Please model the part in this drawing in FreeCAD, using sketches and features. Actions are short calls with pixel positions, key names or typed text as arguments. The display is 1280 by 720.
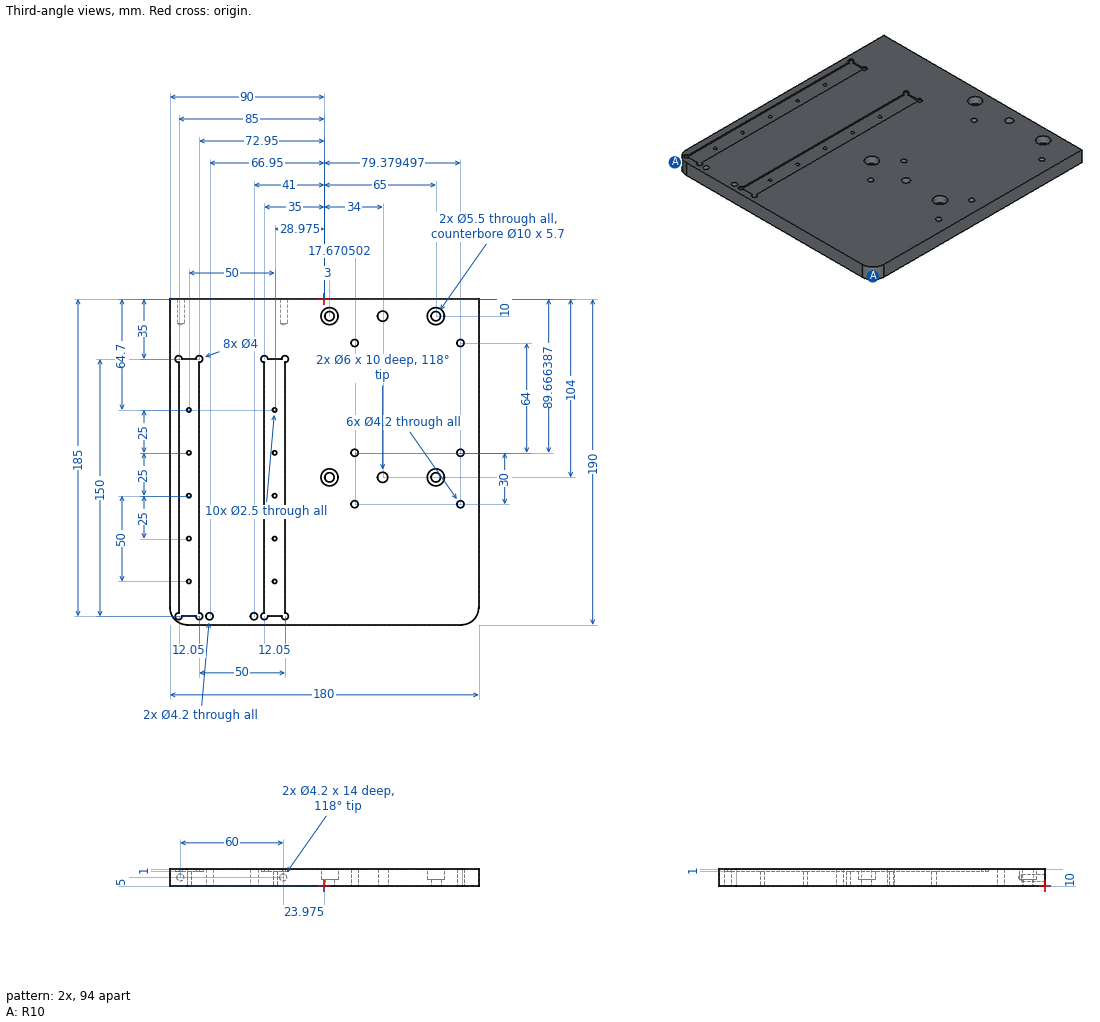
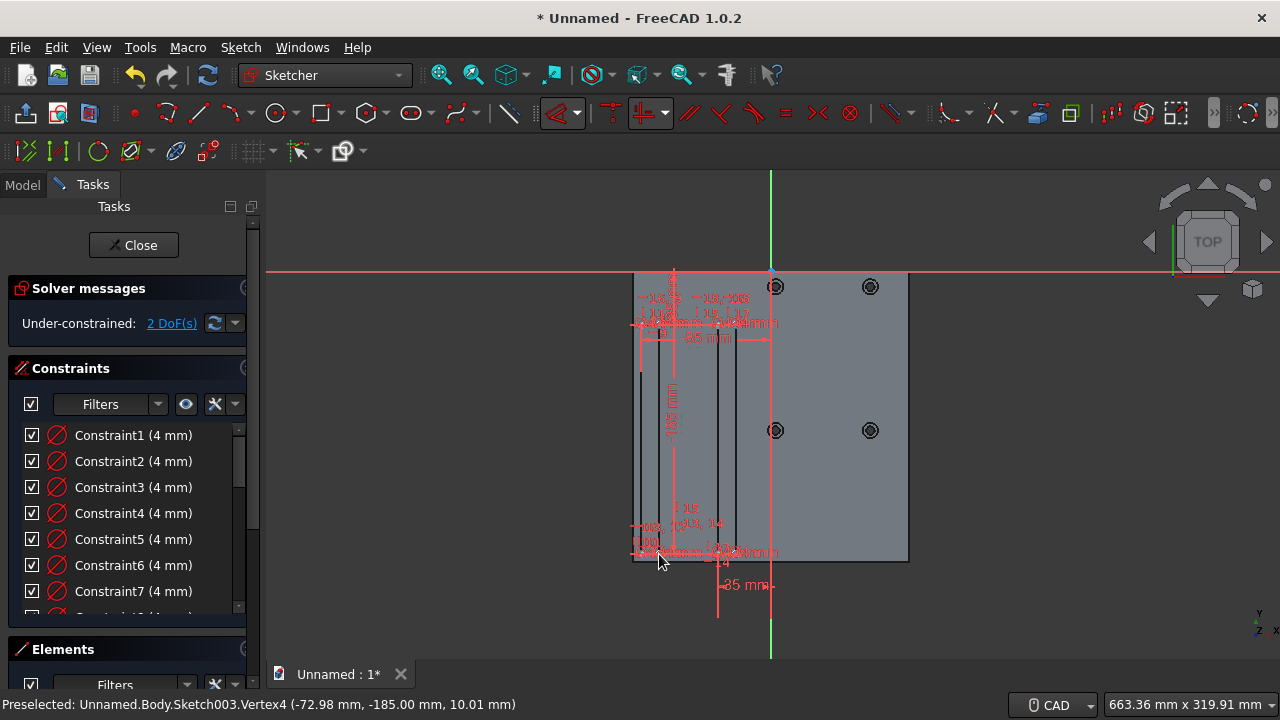
click(735, 554)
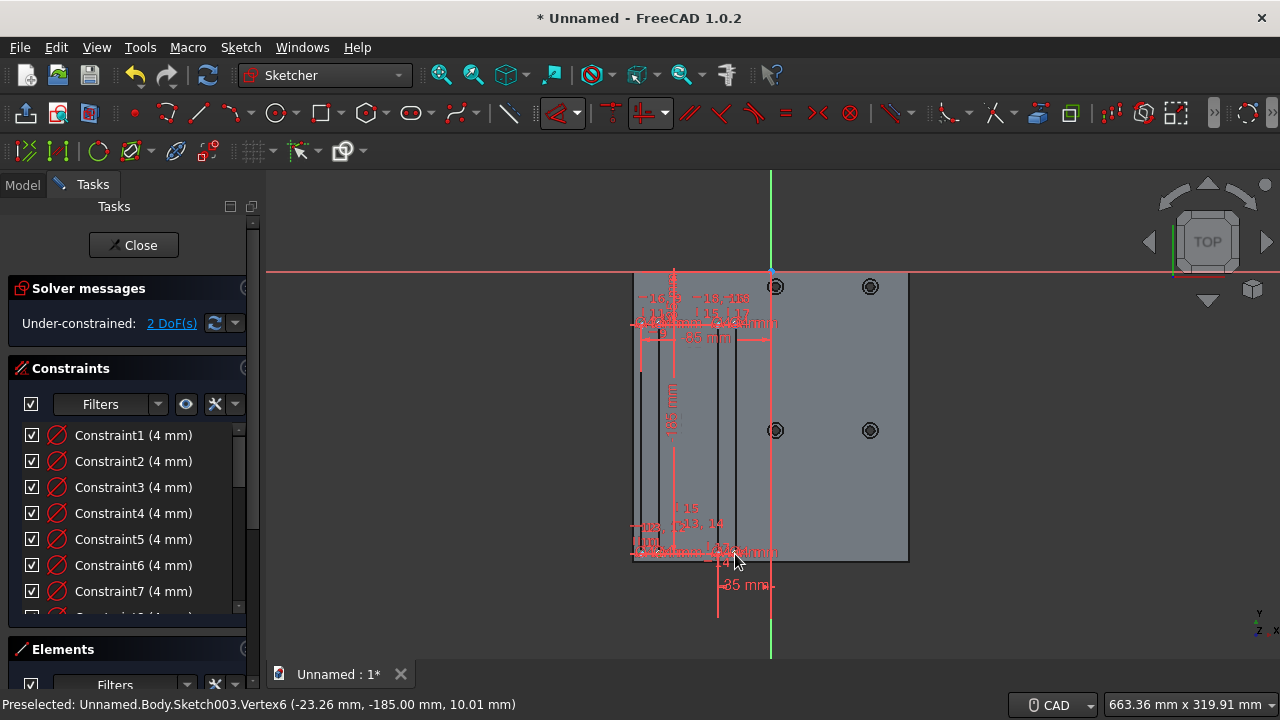
key(l)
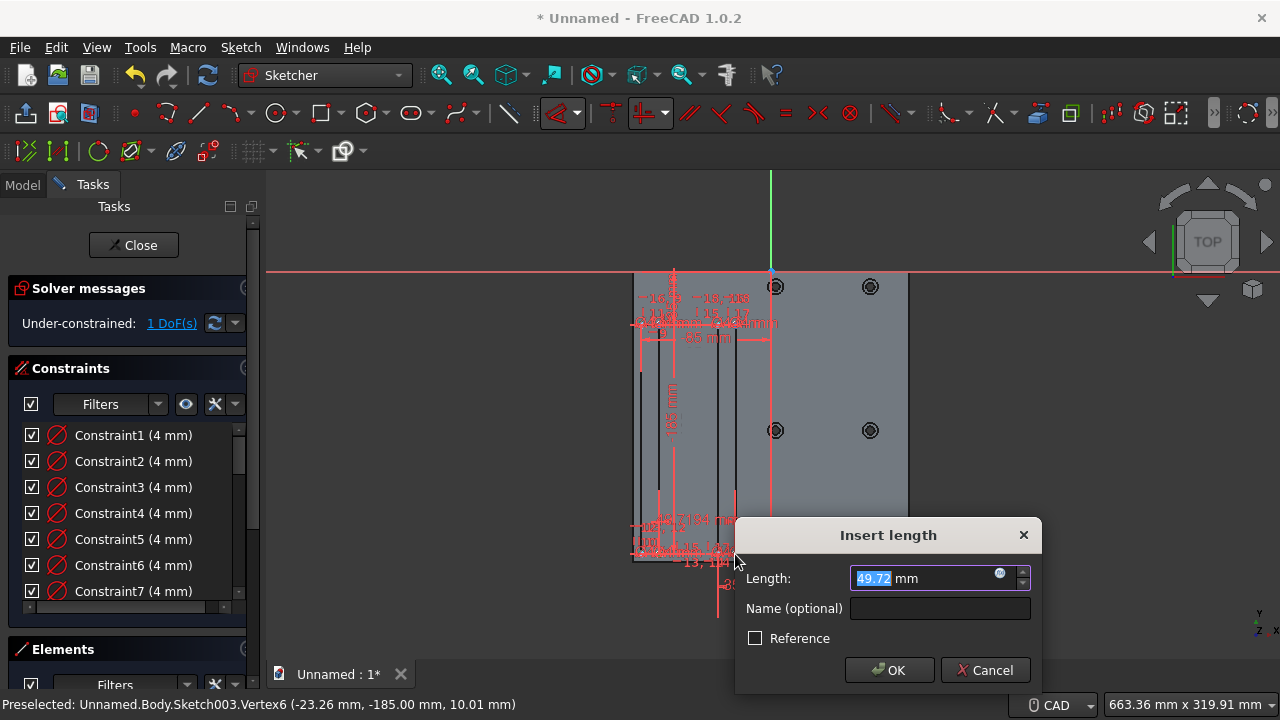
text(50)
key(Return)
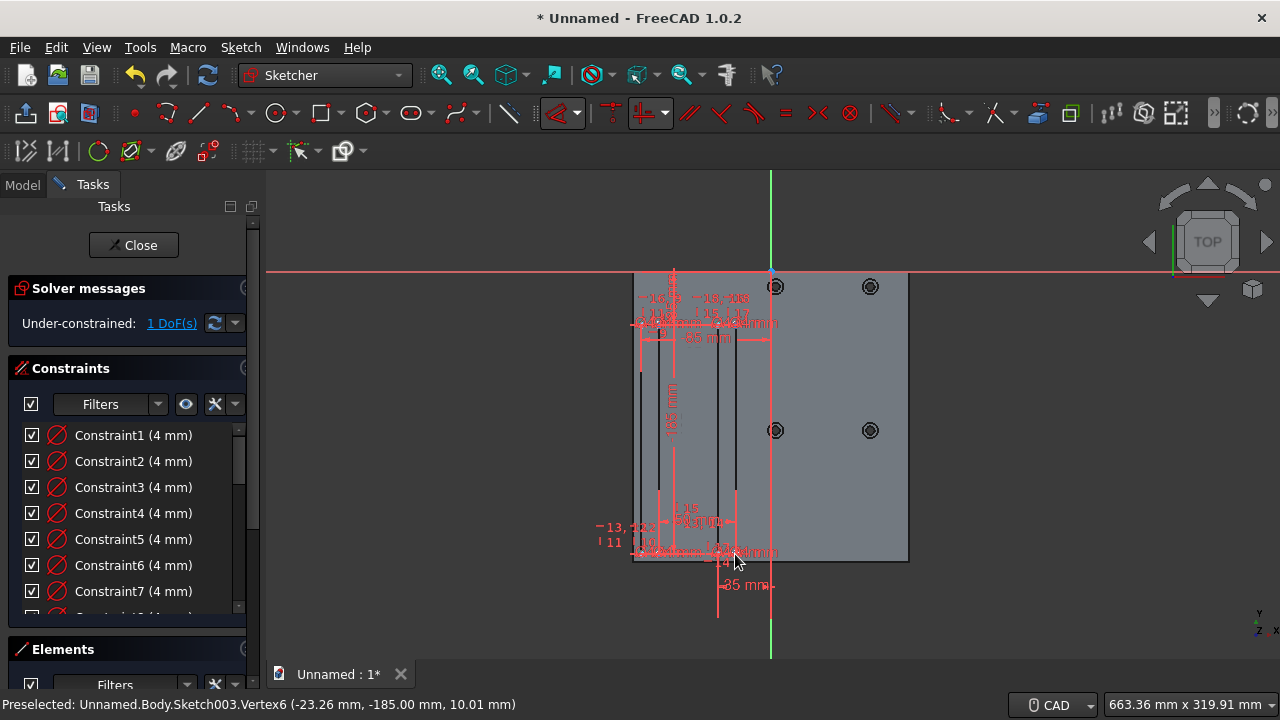
click(659, 325)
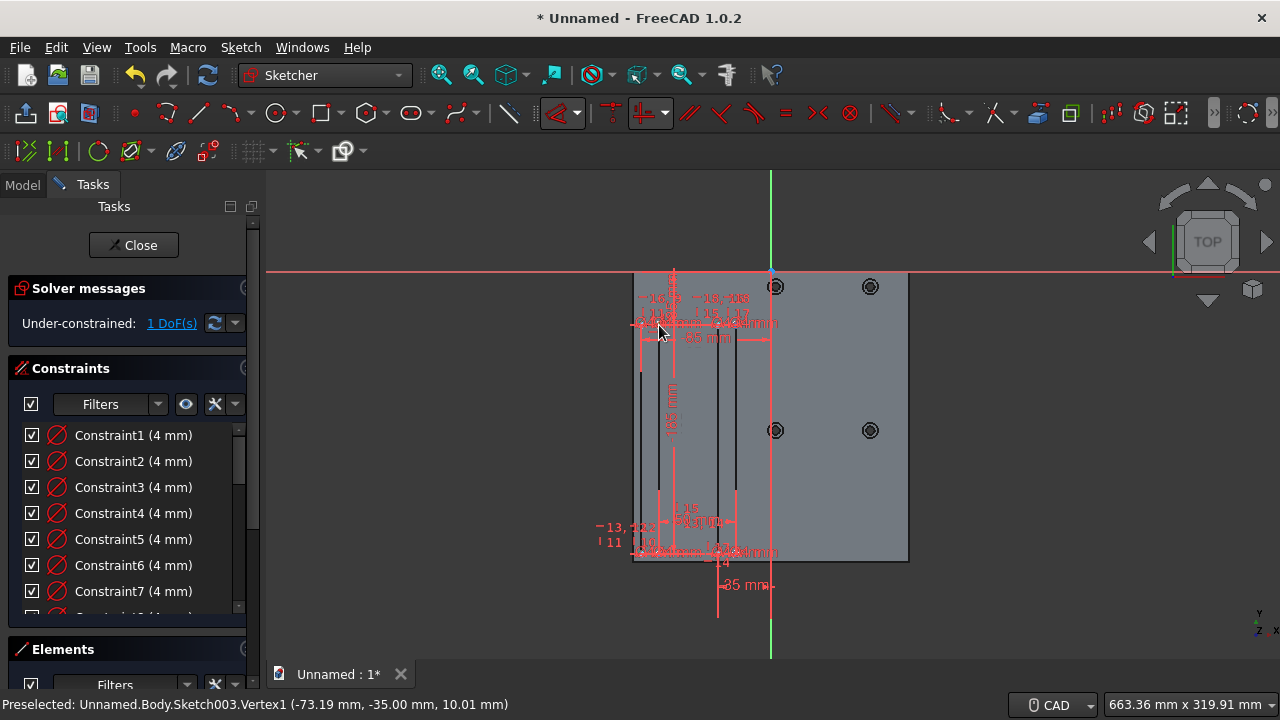
click(580, 114)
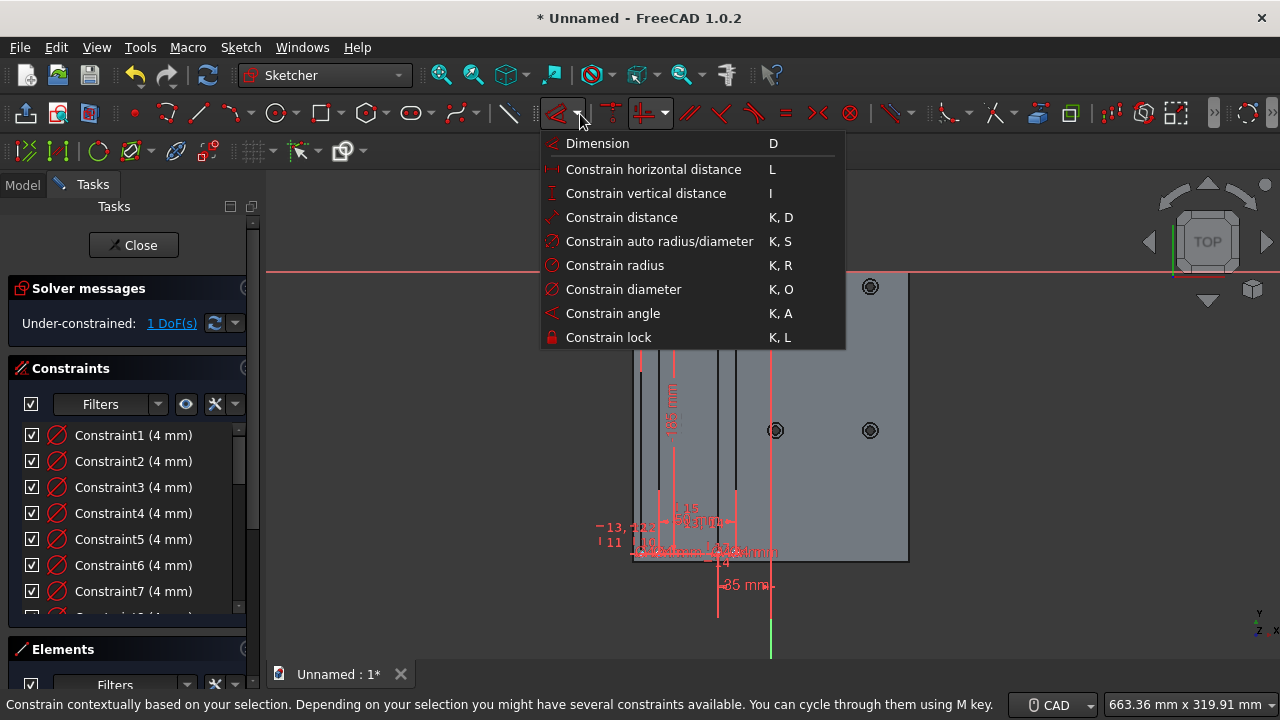
click(693, 169)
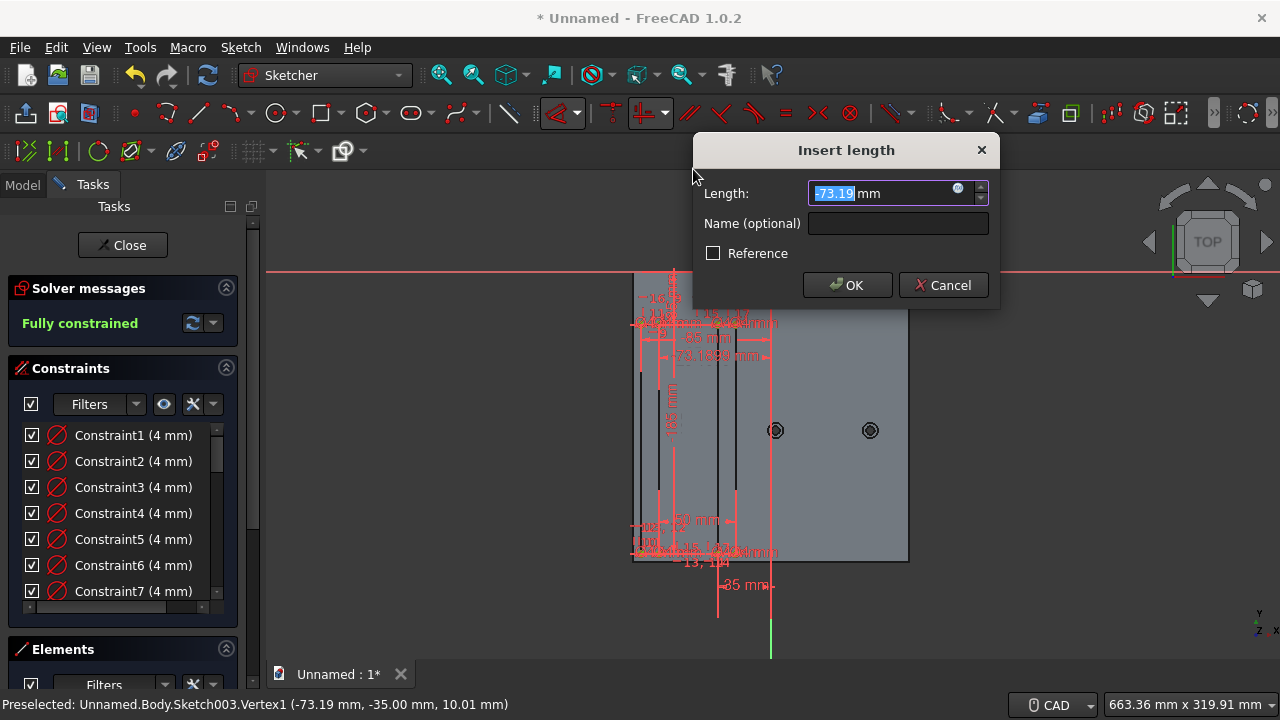
text(-72.95)
key(Return)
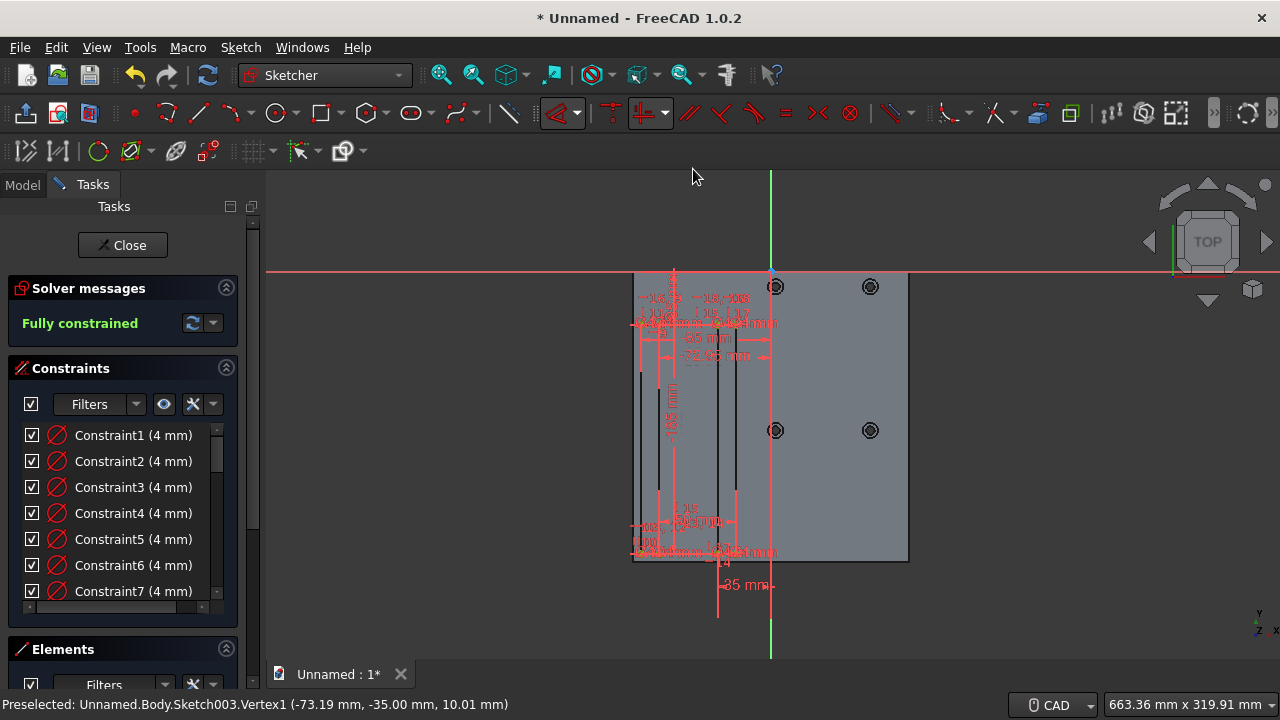
click(123, 245)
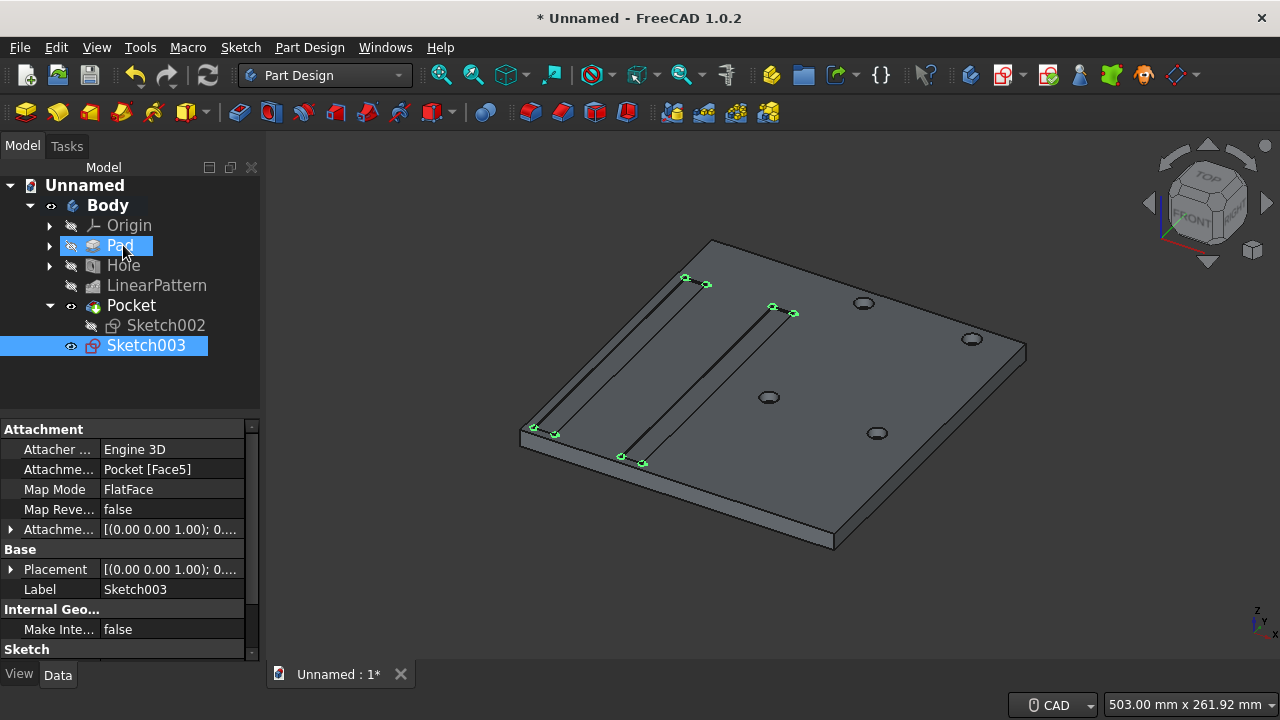
click(240, 112)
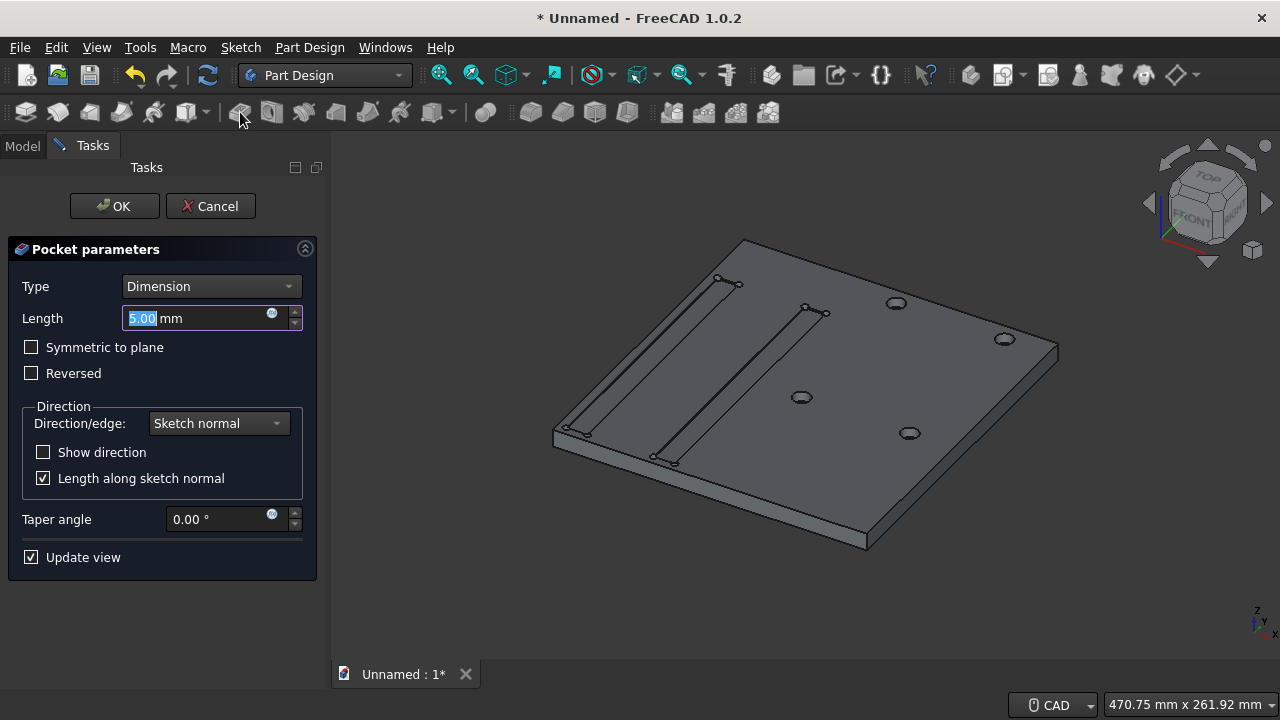
text(1)
key(Tab)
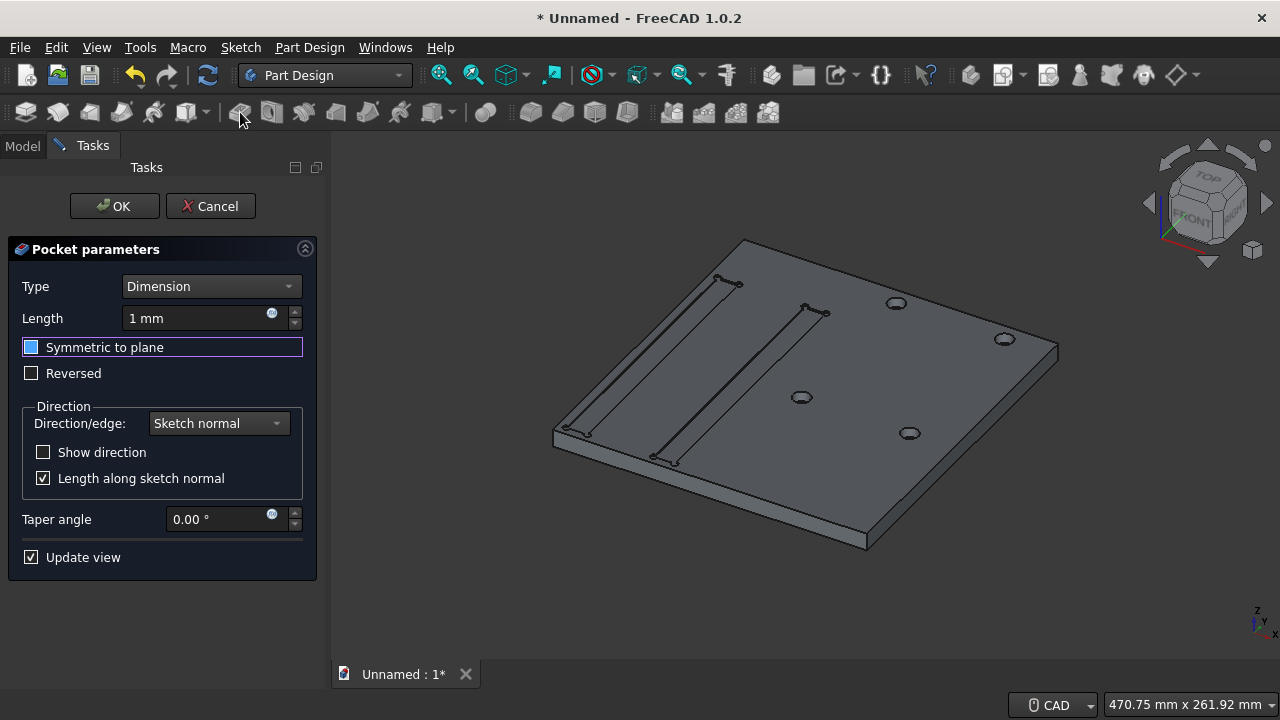
click(115, 206)